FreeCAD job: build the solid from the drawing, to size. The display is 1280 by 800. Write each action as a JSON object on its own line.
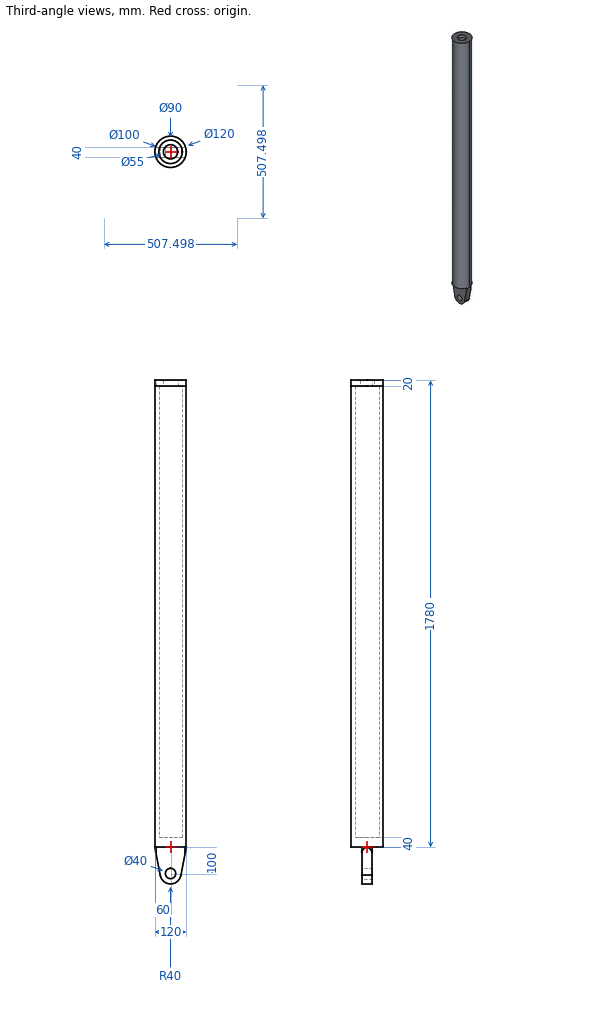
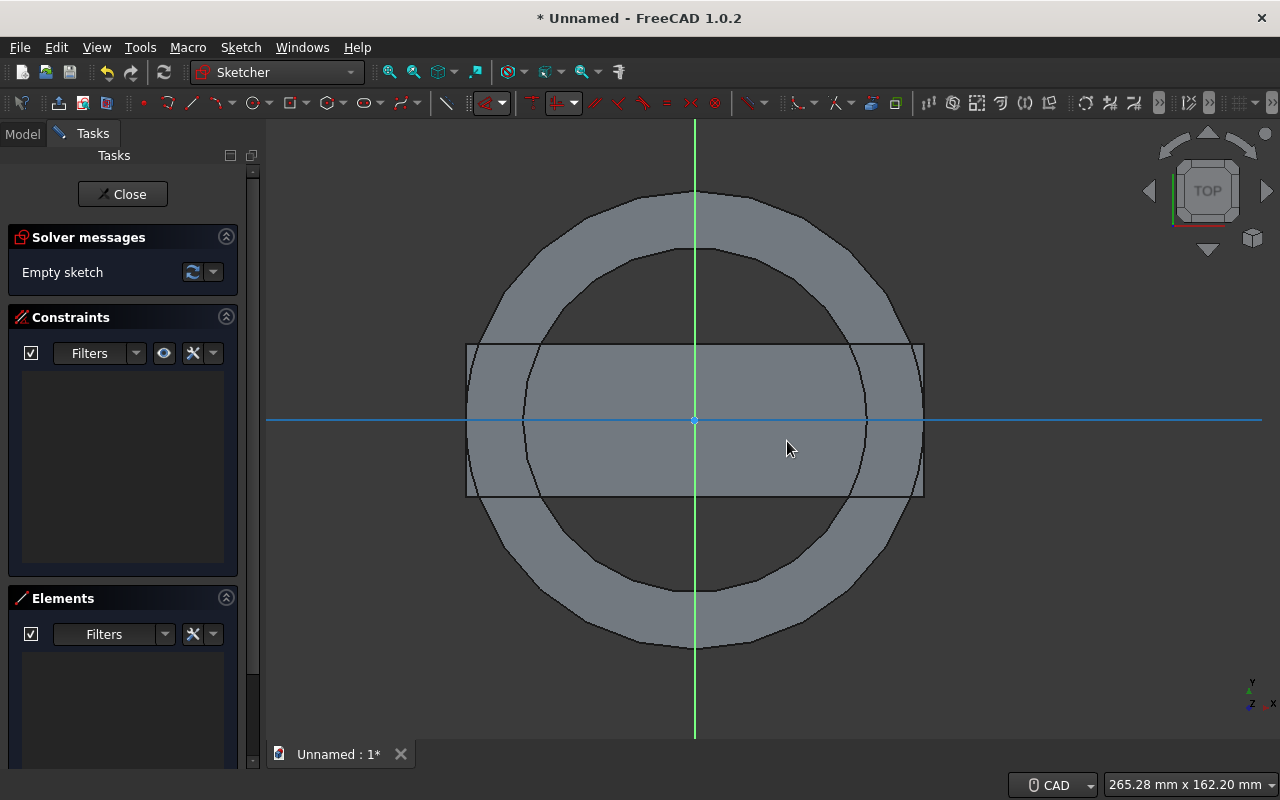
{"action": "key", "text": "g c"}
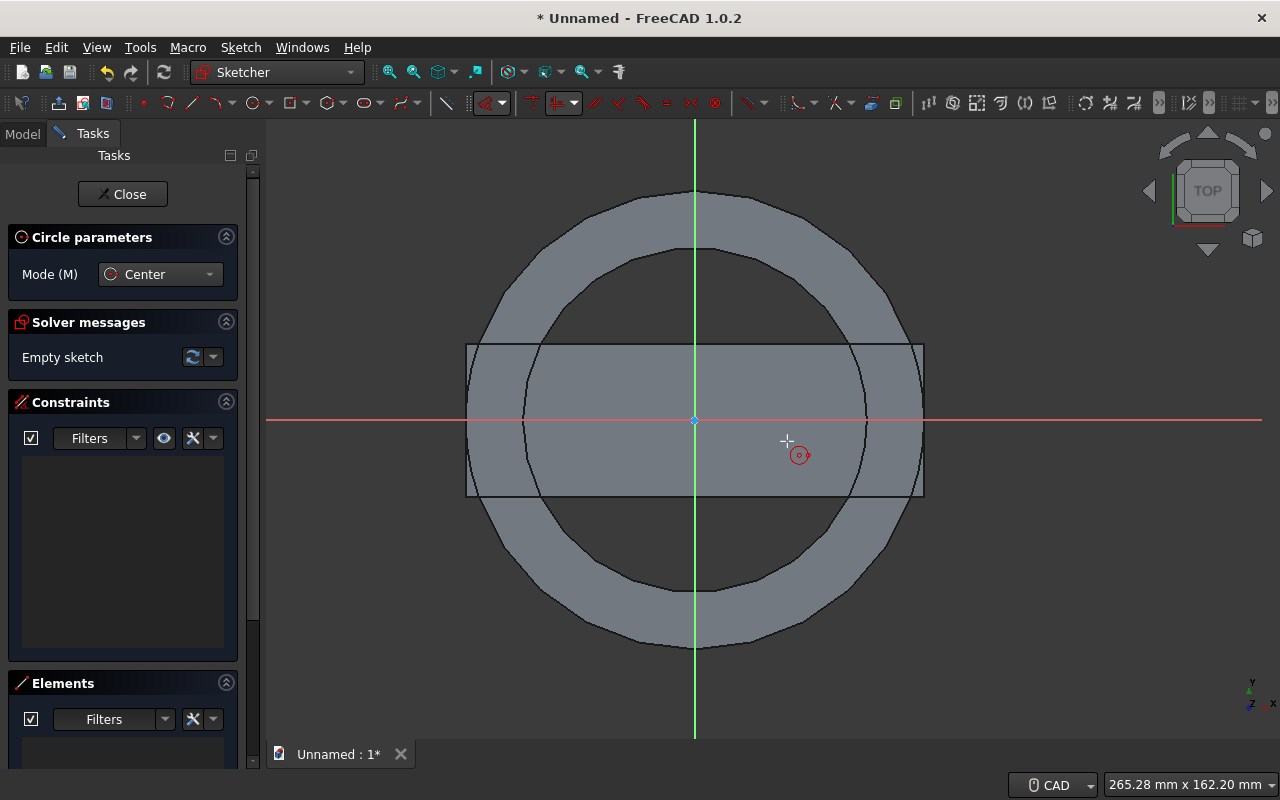
{"action": "left_click", "coordinate": [695, 420]}
{"action": "mouse_move", "coordinate": [830, 285]}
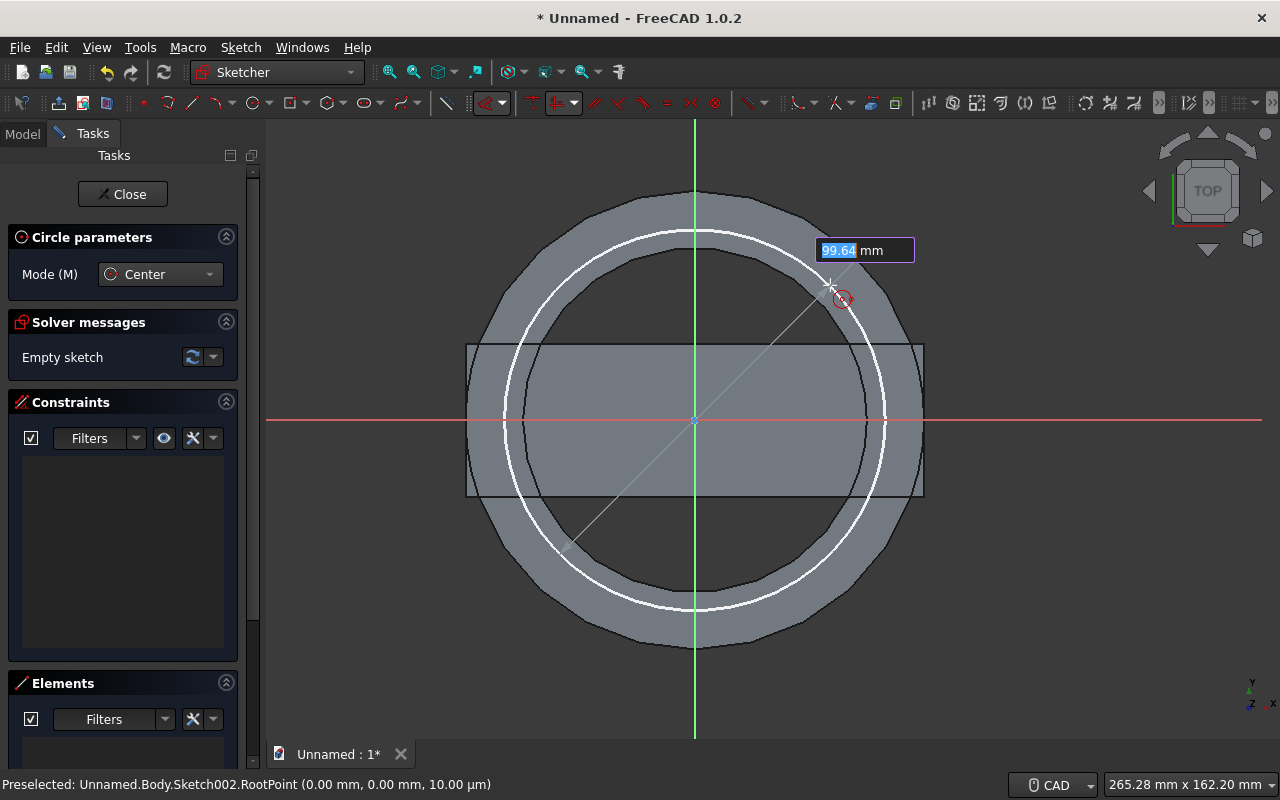
{"action": "type", "text": "100"}
{"action": "key", "text": "Return"}
{"action": "key", "text": "Escape"}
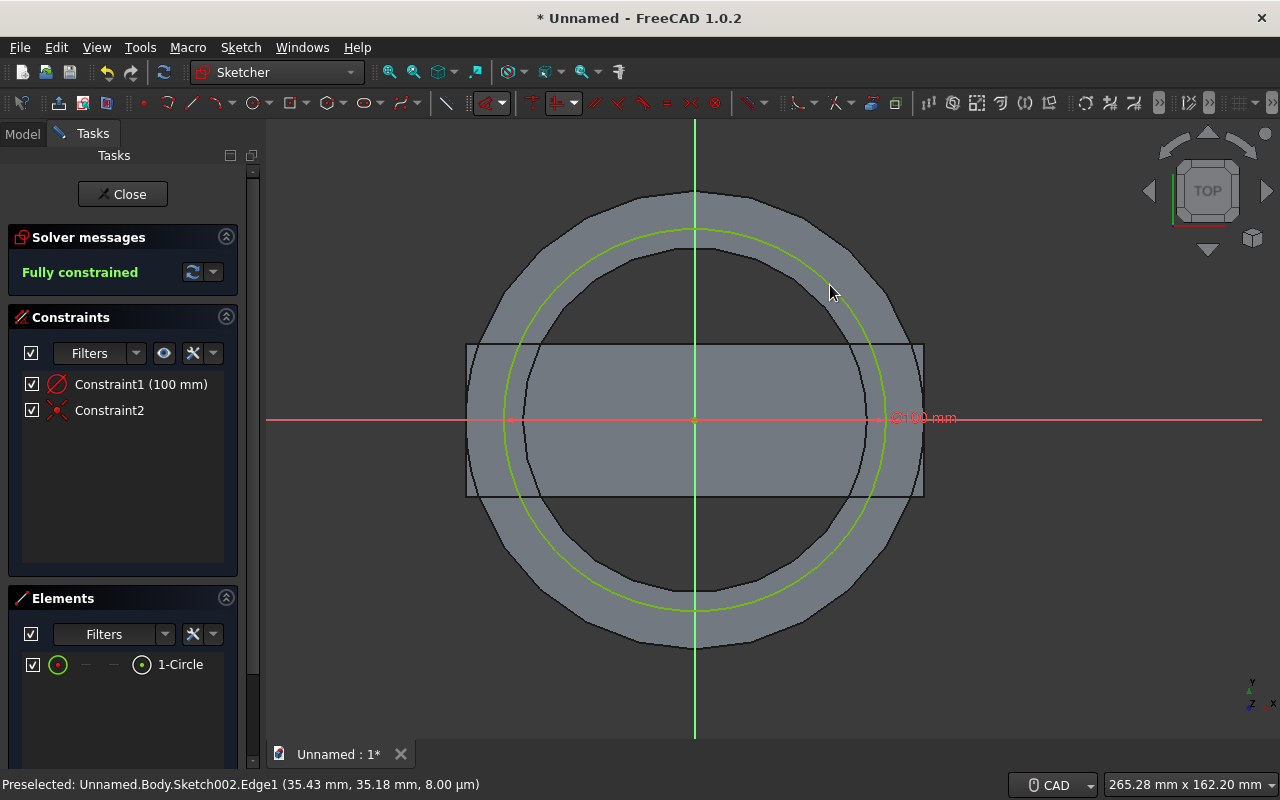
{"action": "left_click", "coordinate": [123, 194]}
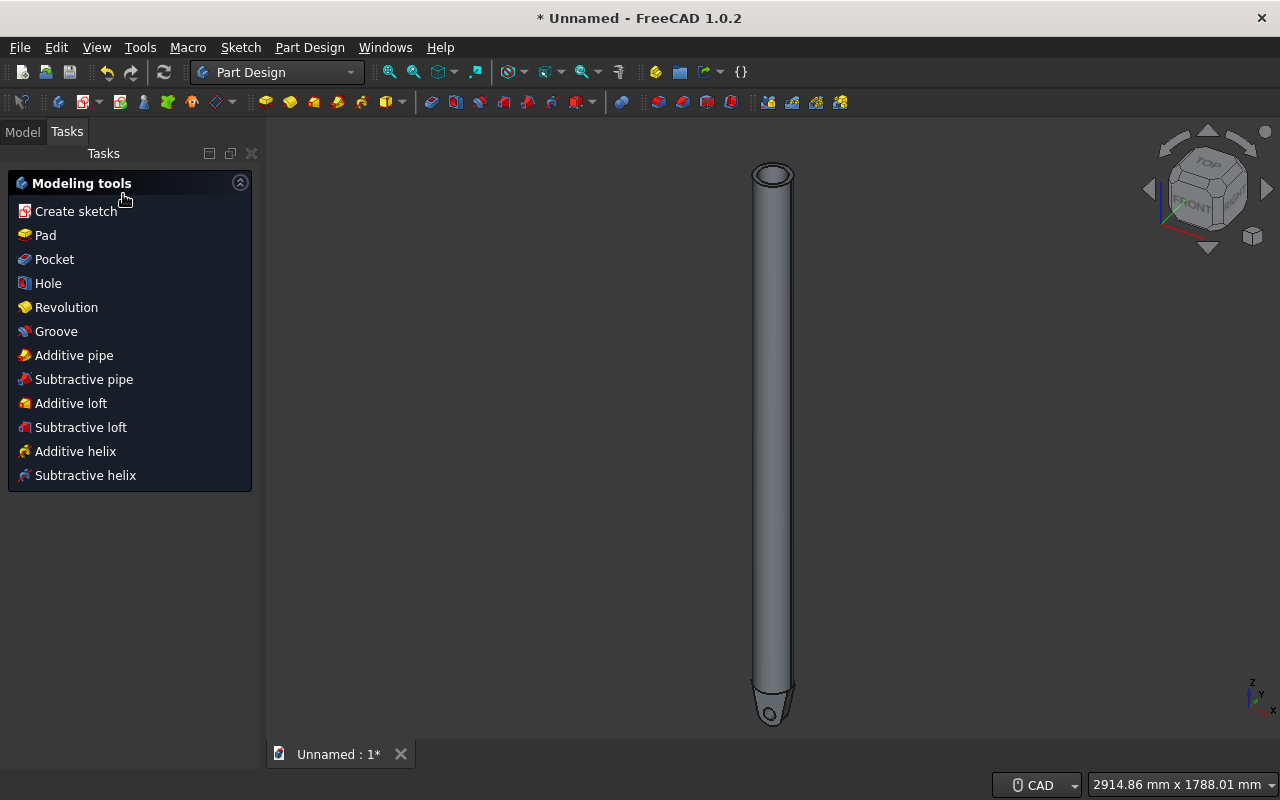
{"action": "left_click", "coordinate": [266, 102]}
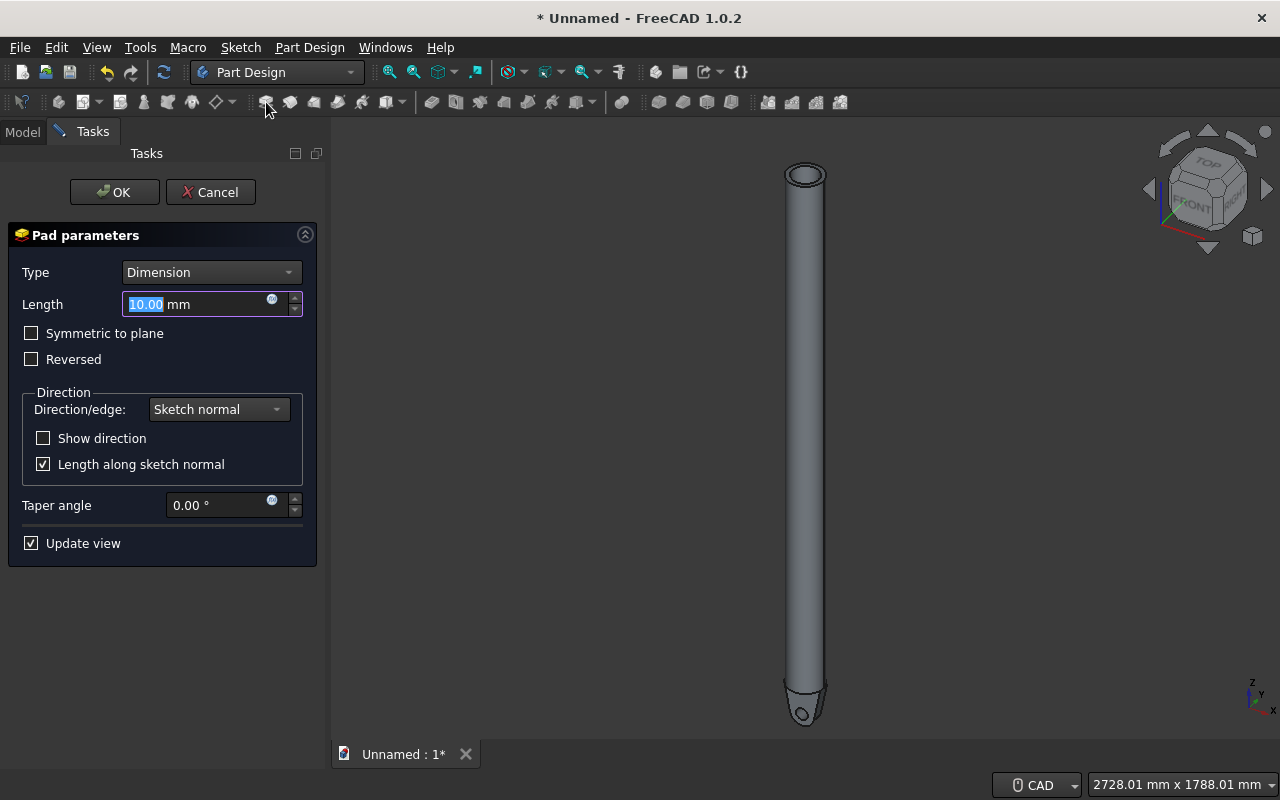
{"action": "type", "text": "40"}
{"action": "key", "text": "Tab"}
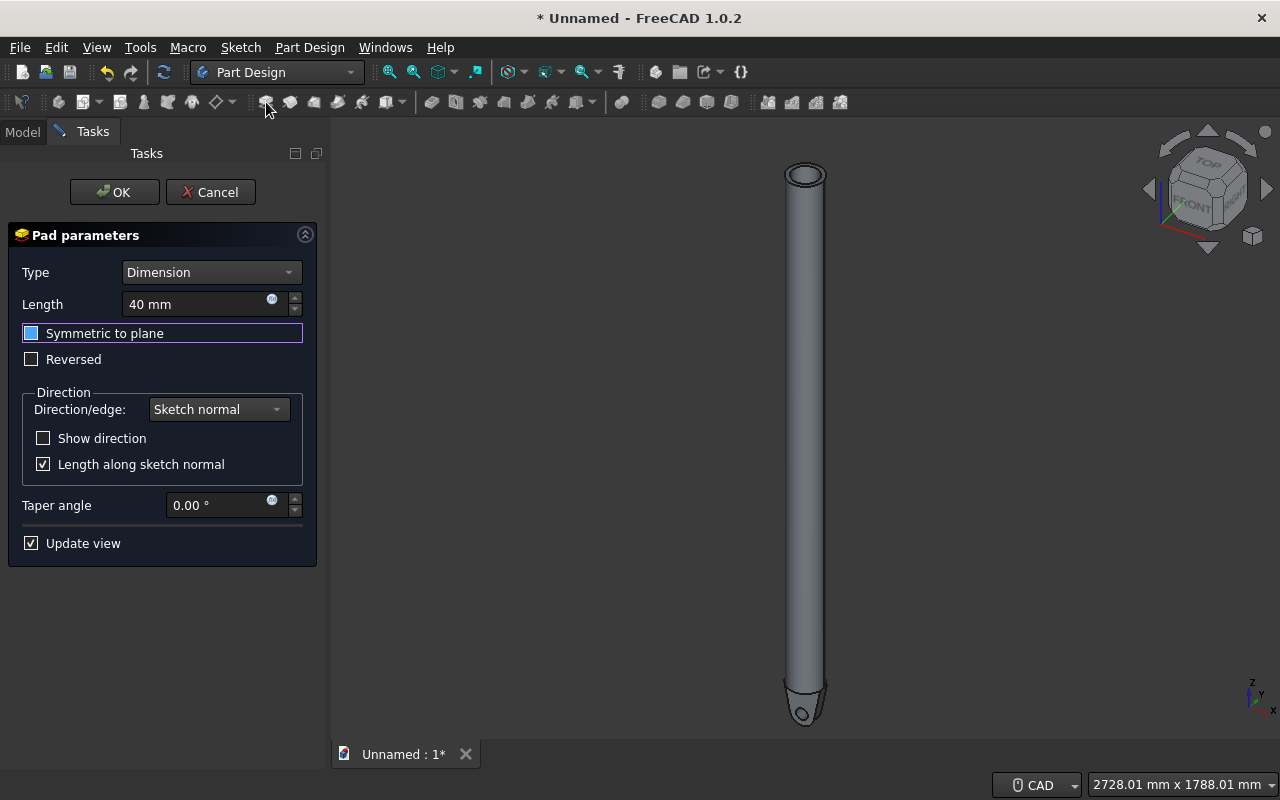
{"action": "left_click", "coordinate": [115, 192]}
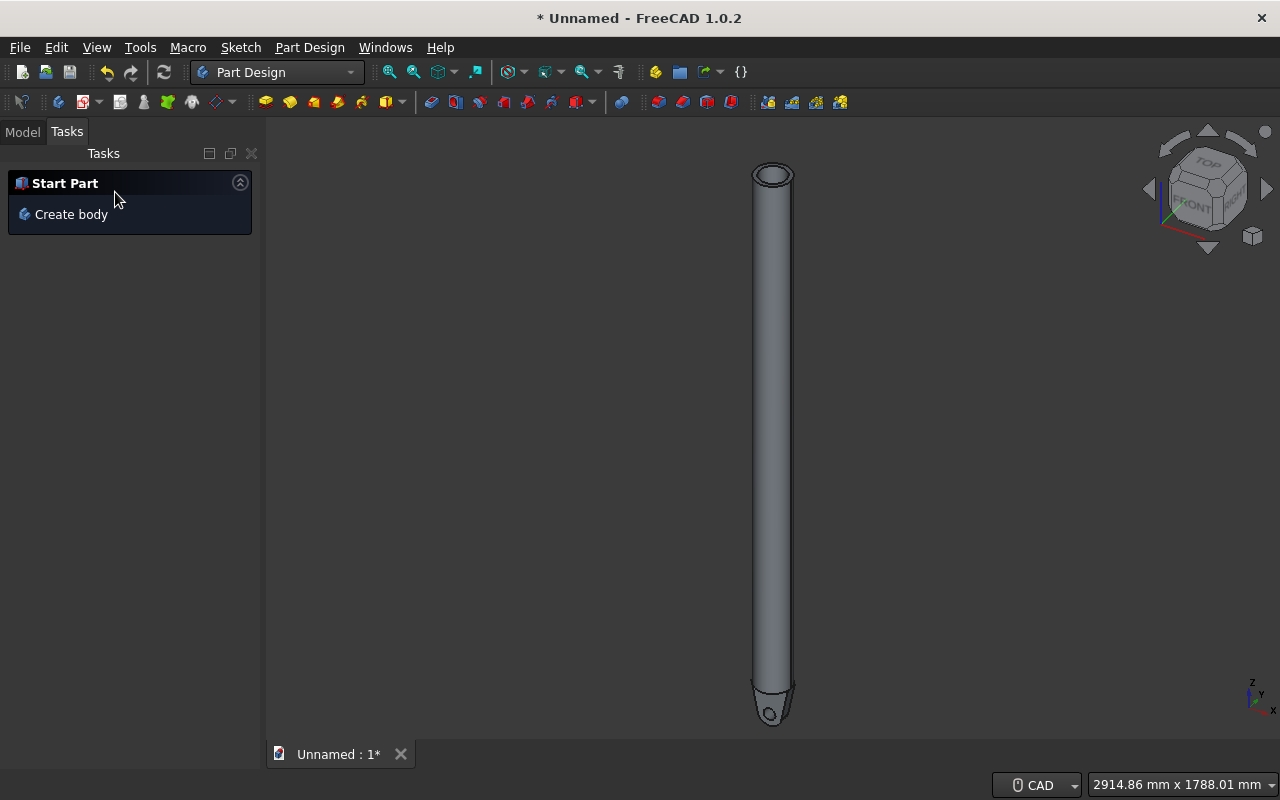
{"action": "left_click", "coordinate": [84, 102]}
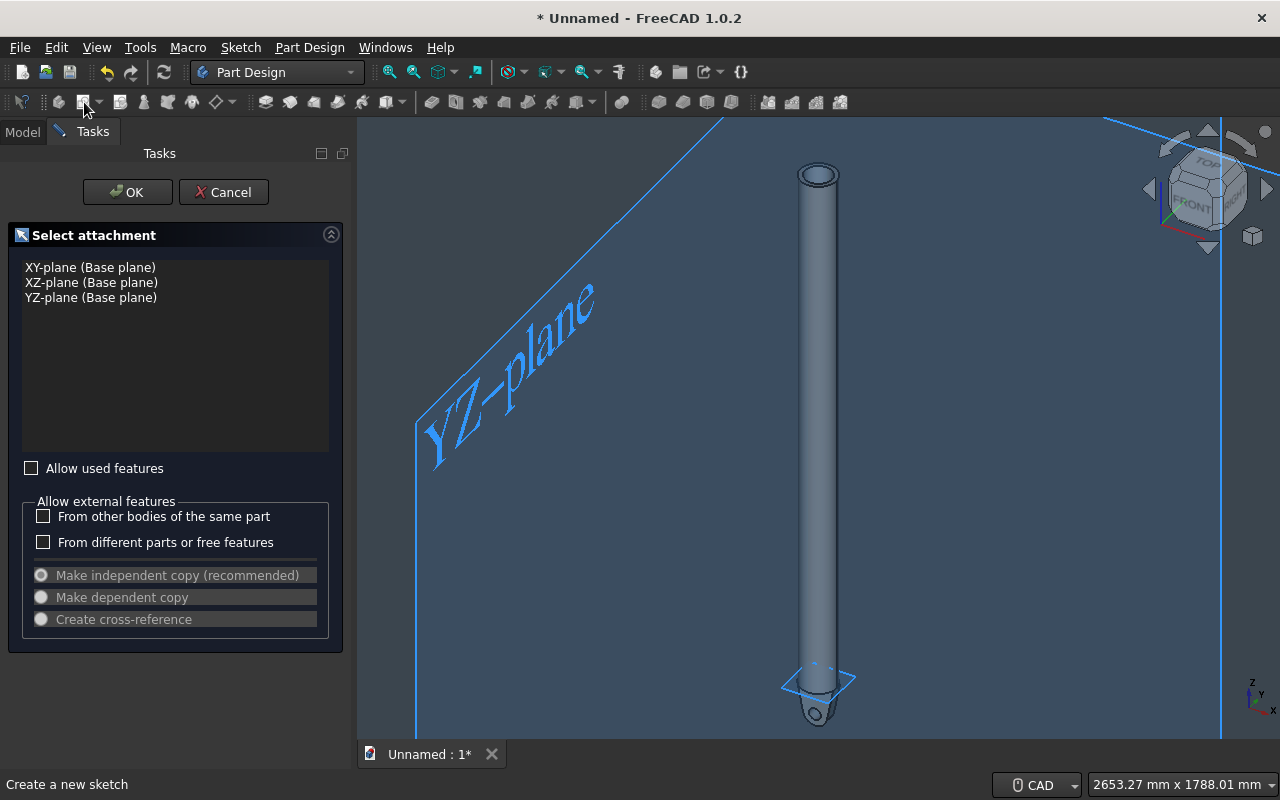
{"action": "left_click", "coordinate": [82, 268]}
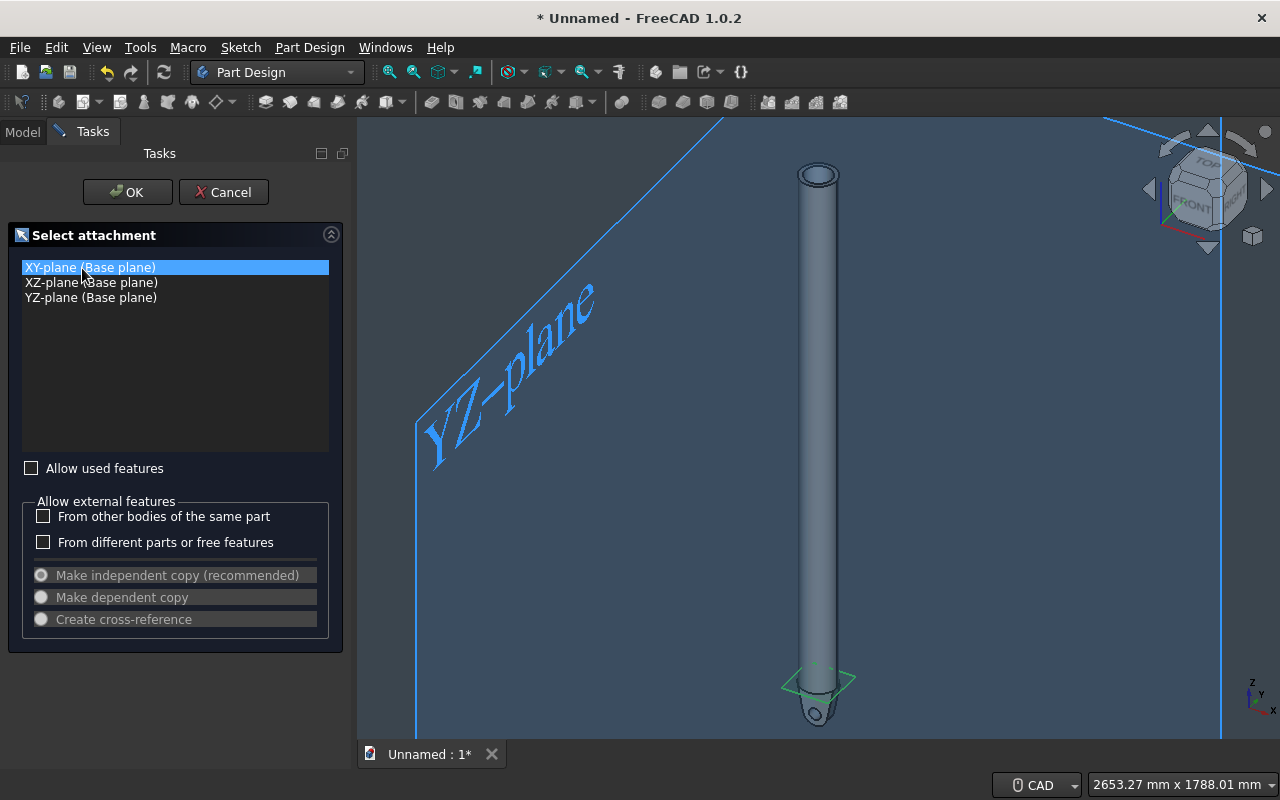
{"action": "left_click", "coordinate": [128, 192]}